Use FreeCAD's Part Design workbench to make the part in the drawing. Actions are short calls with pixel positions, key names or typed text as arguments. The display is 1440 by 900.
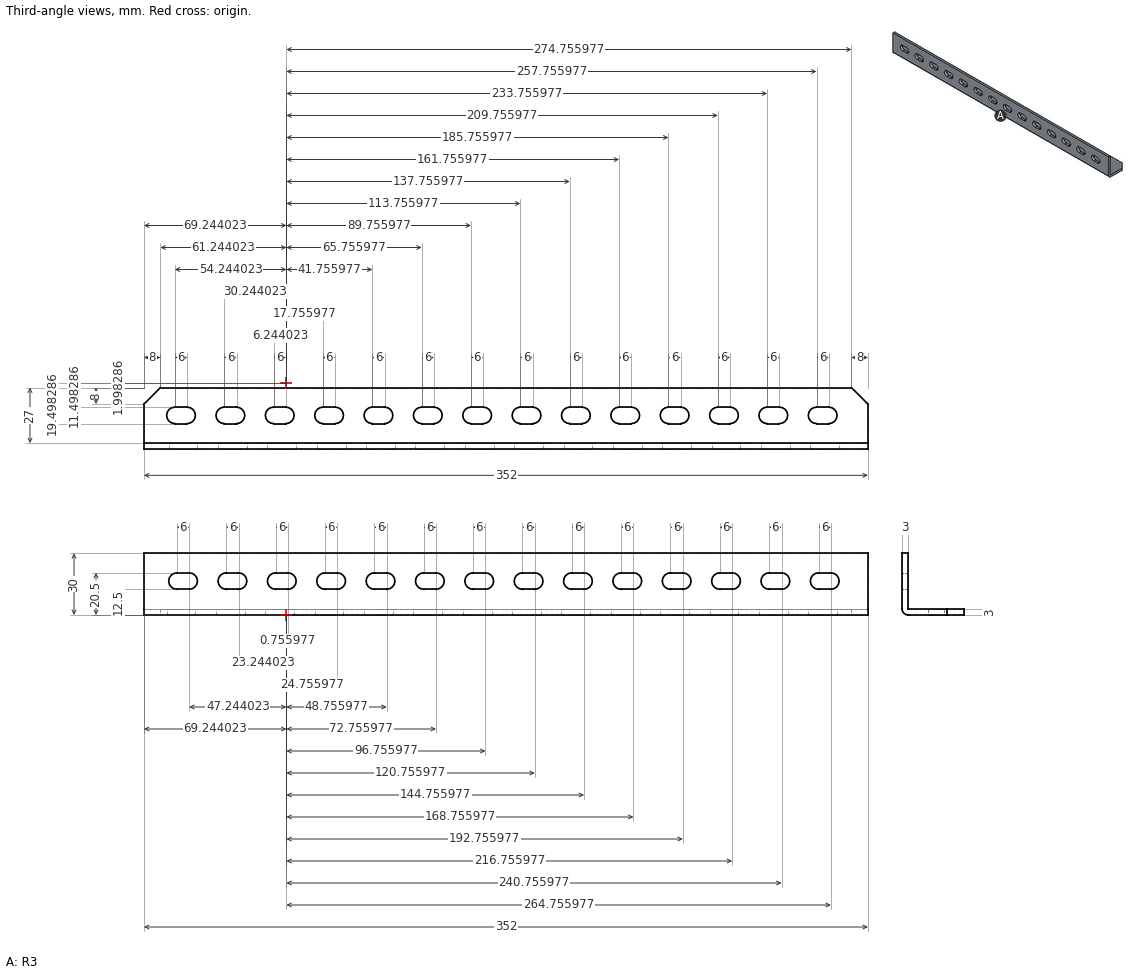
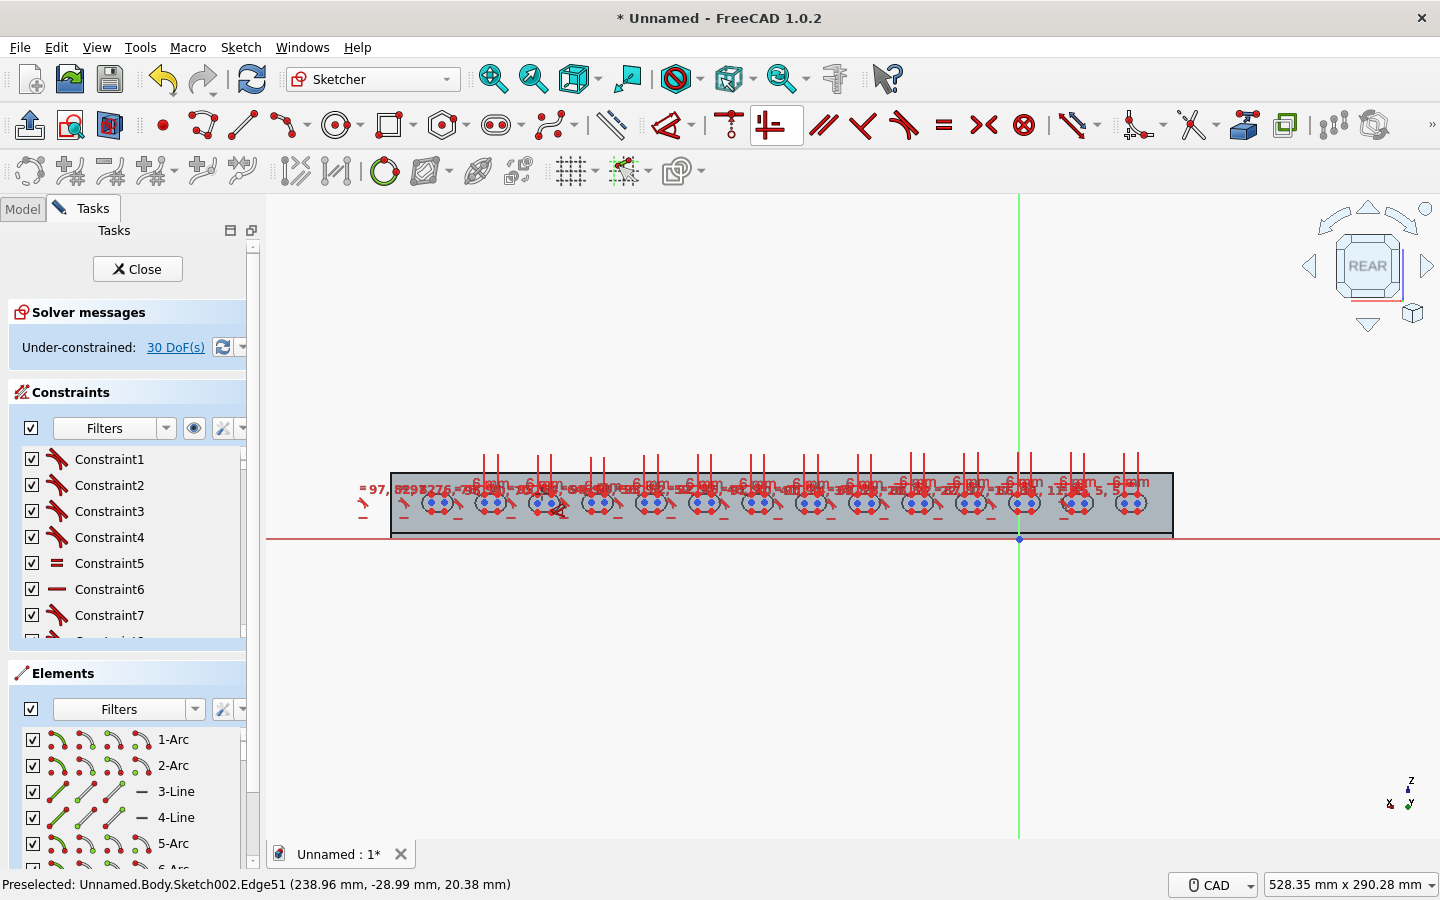
scroll(435, 494, up, 7)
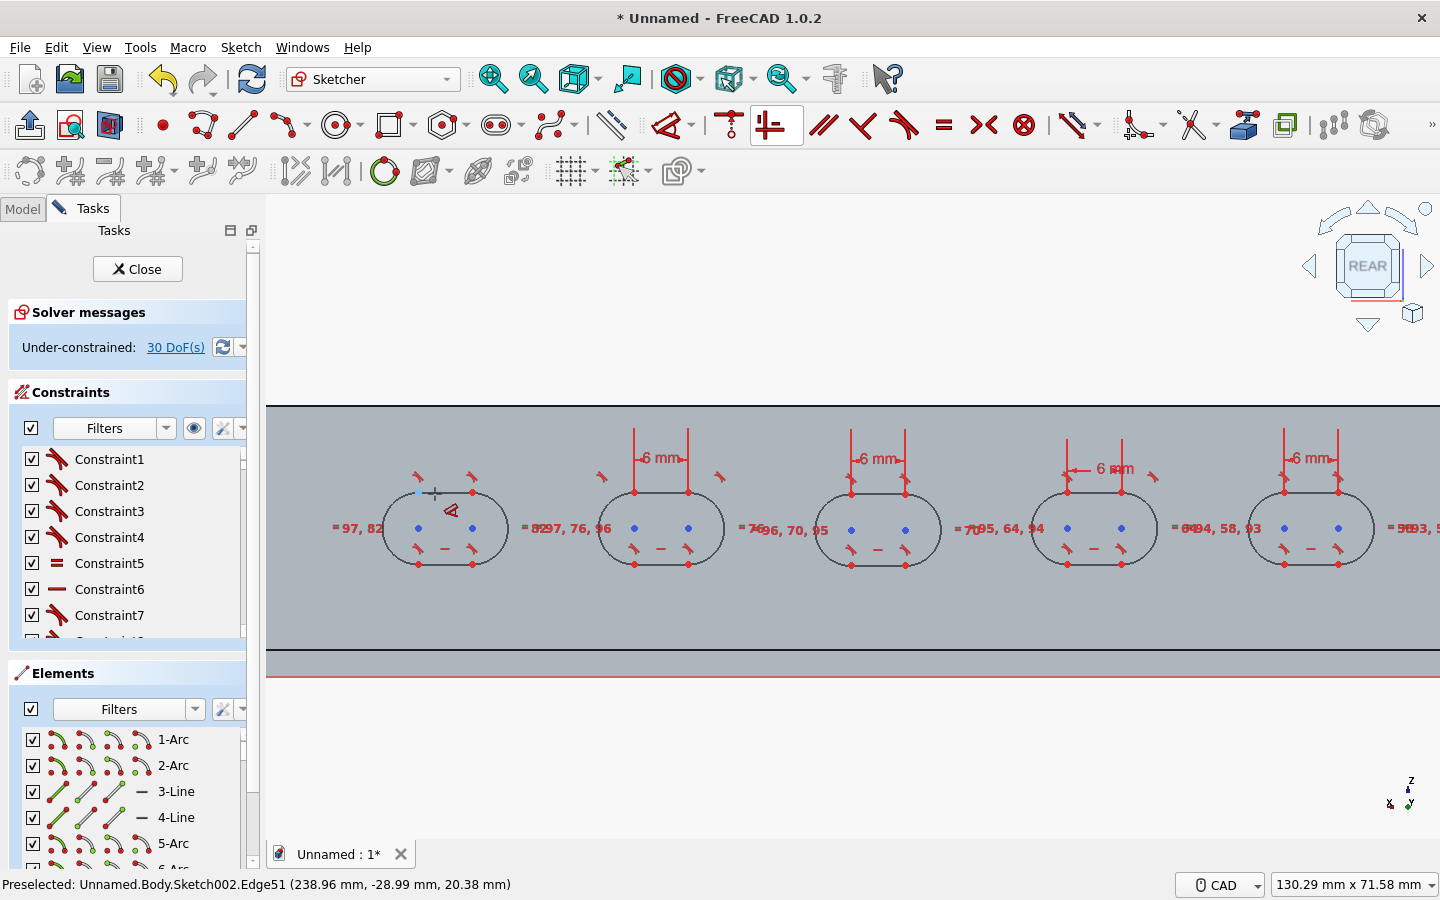
click(434, 493)
click(445, 459)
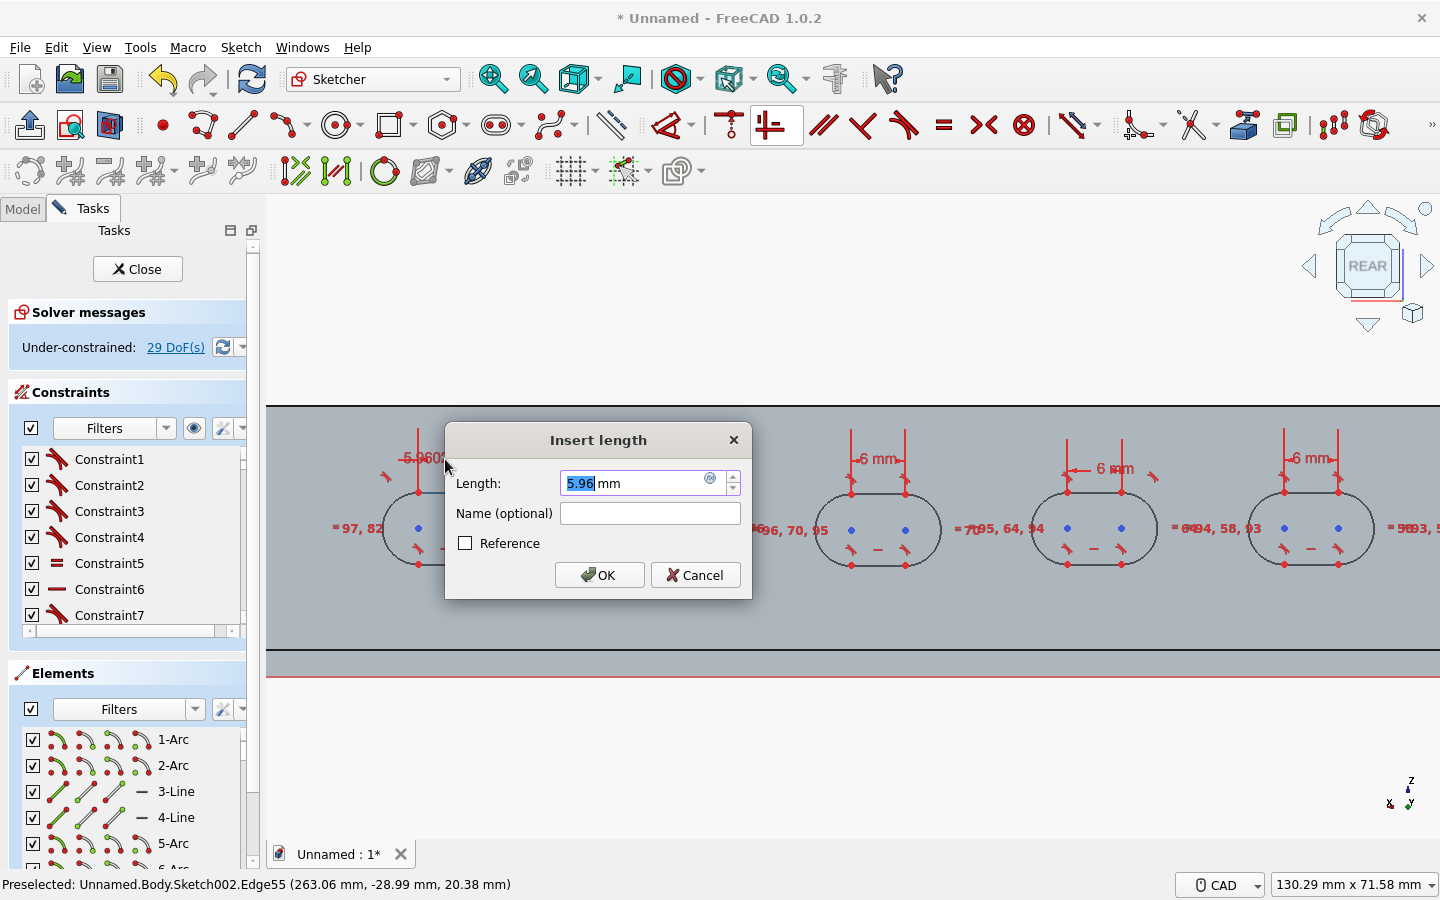
text(6)
key(Return)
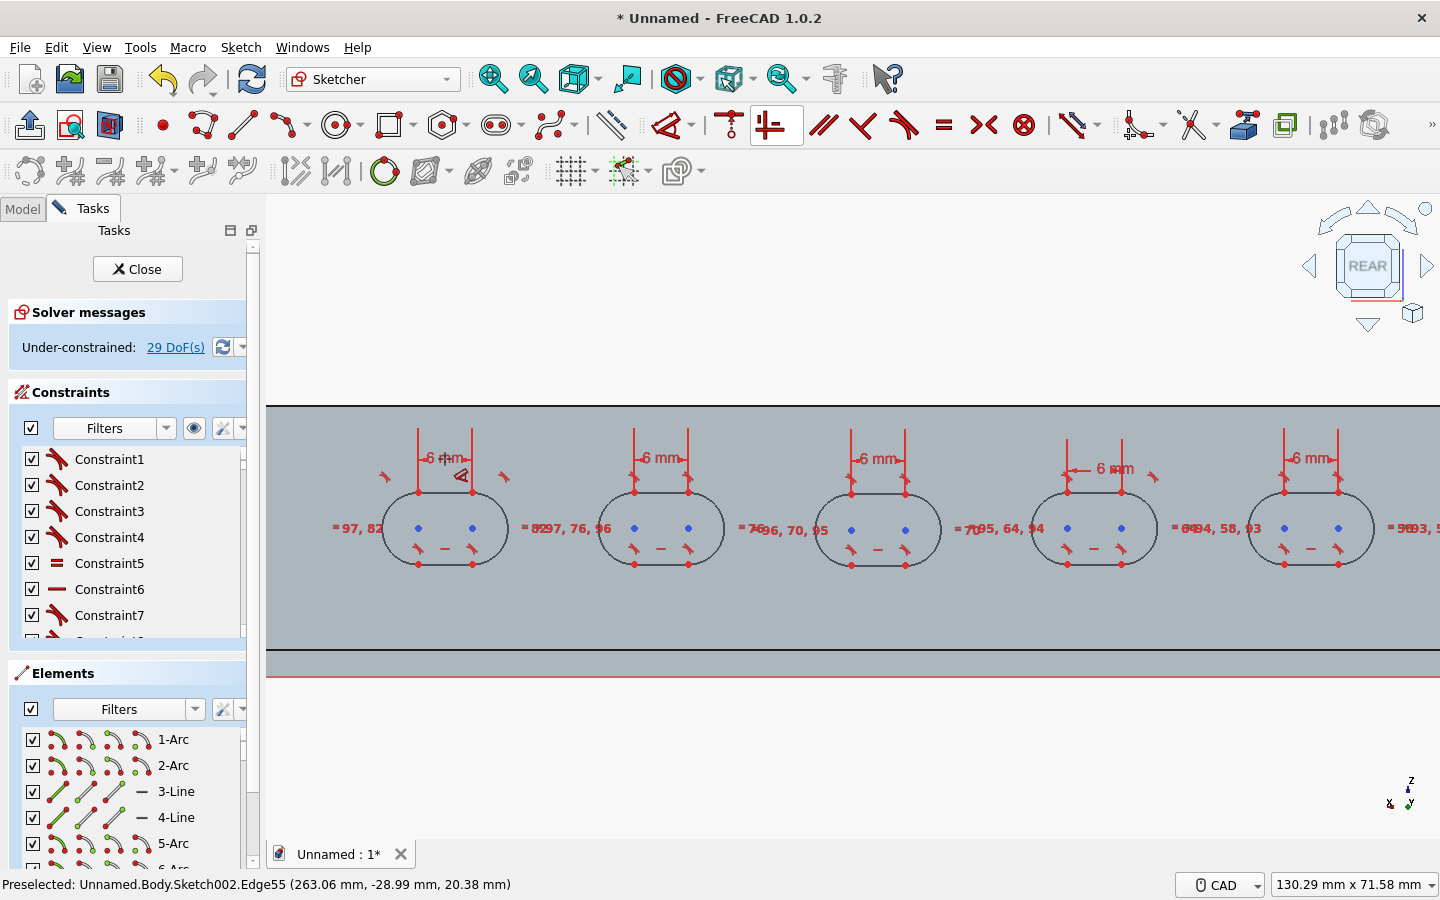
scroll(435, 494, down, 7)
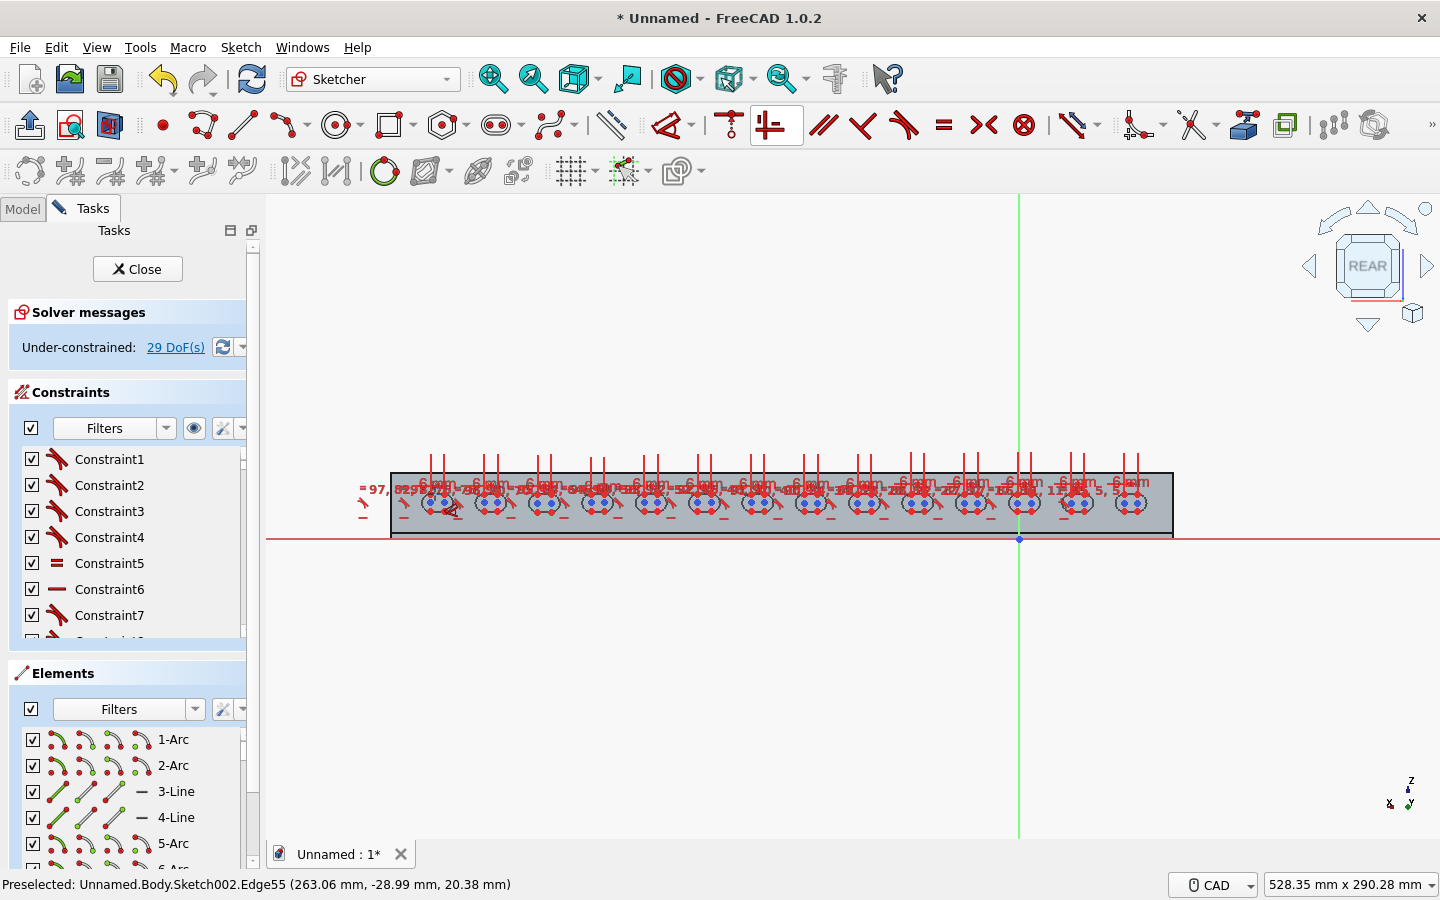
scroll(1124, 494, up, 2)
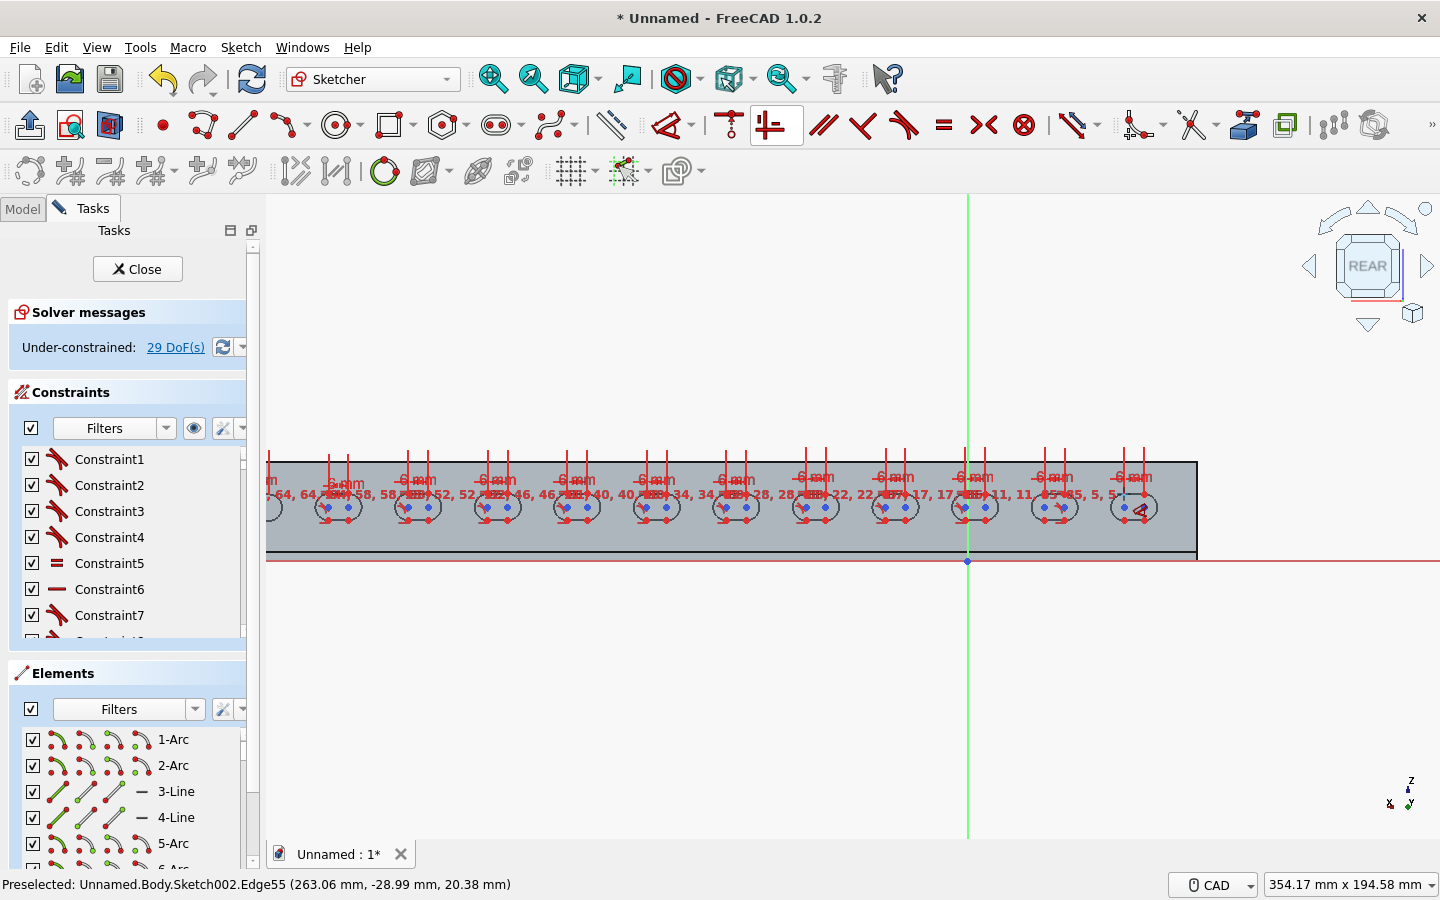
click(1124, 494)
click(1158, 543)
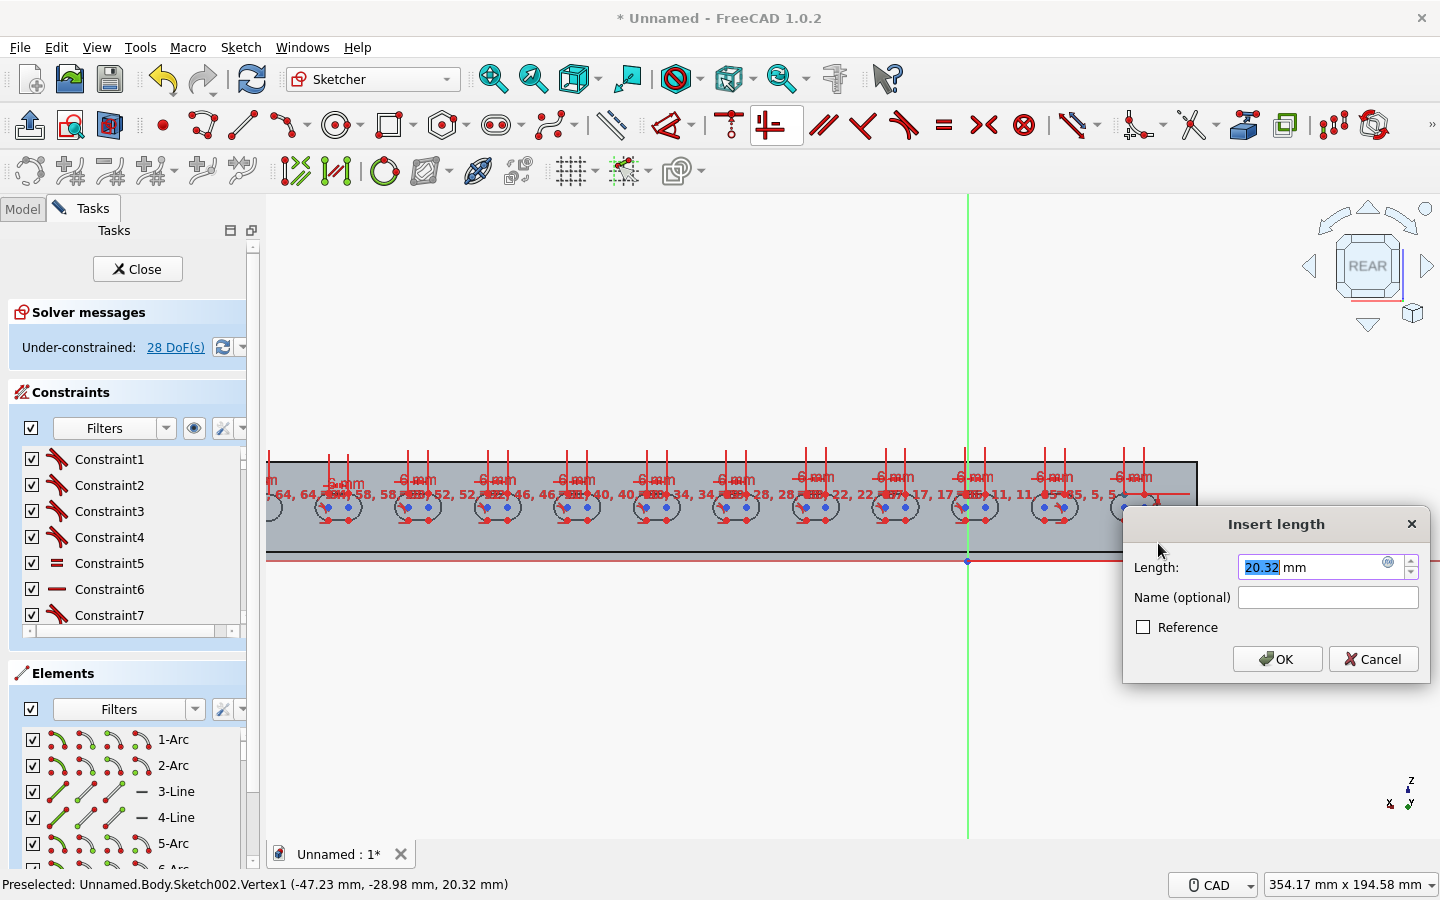
text(20.5)
key(Return)